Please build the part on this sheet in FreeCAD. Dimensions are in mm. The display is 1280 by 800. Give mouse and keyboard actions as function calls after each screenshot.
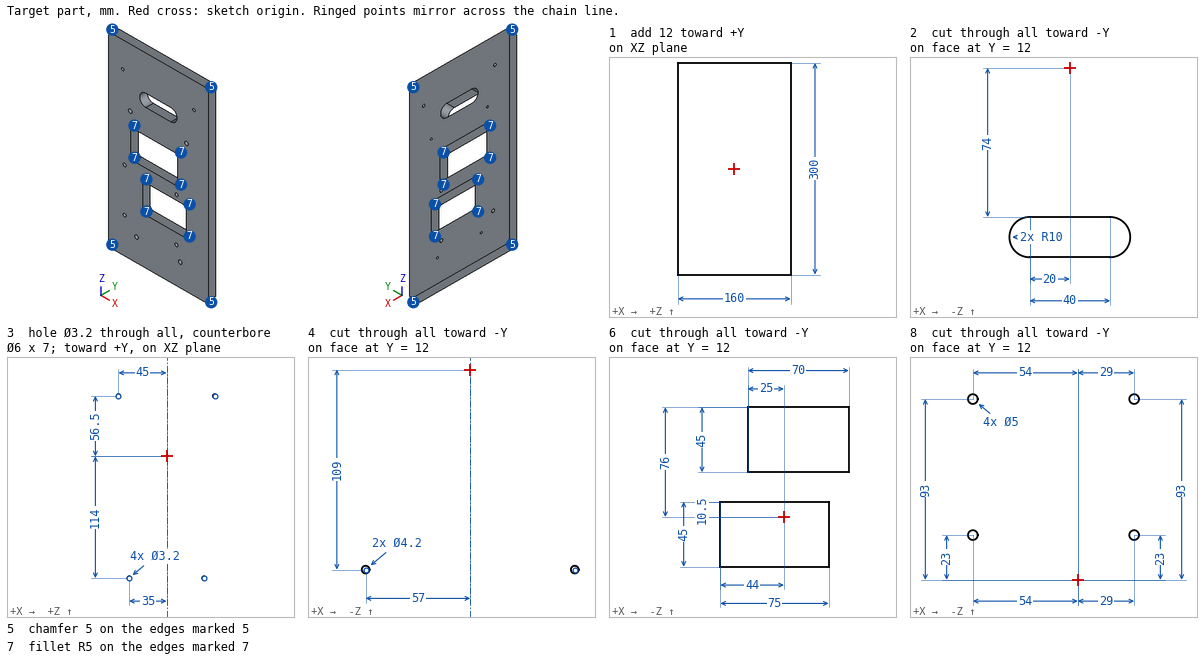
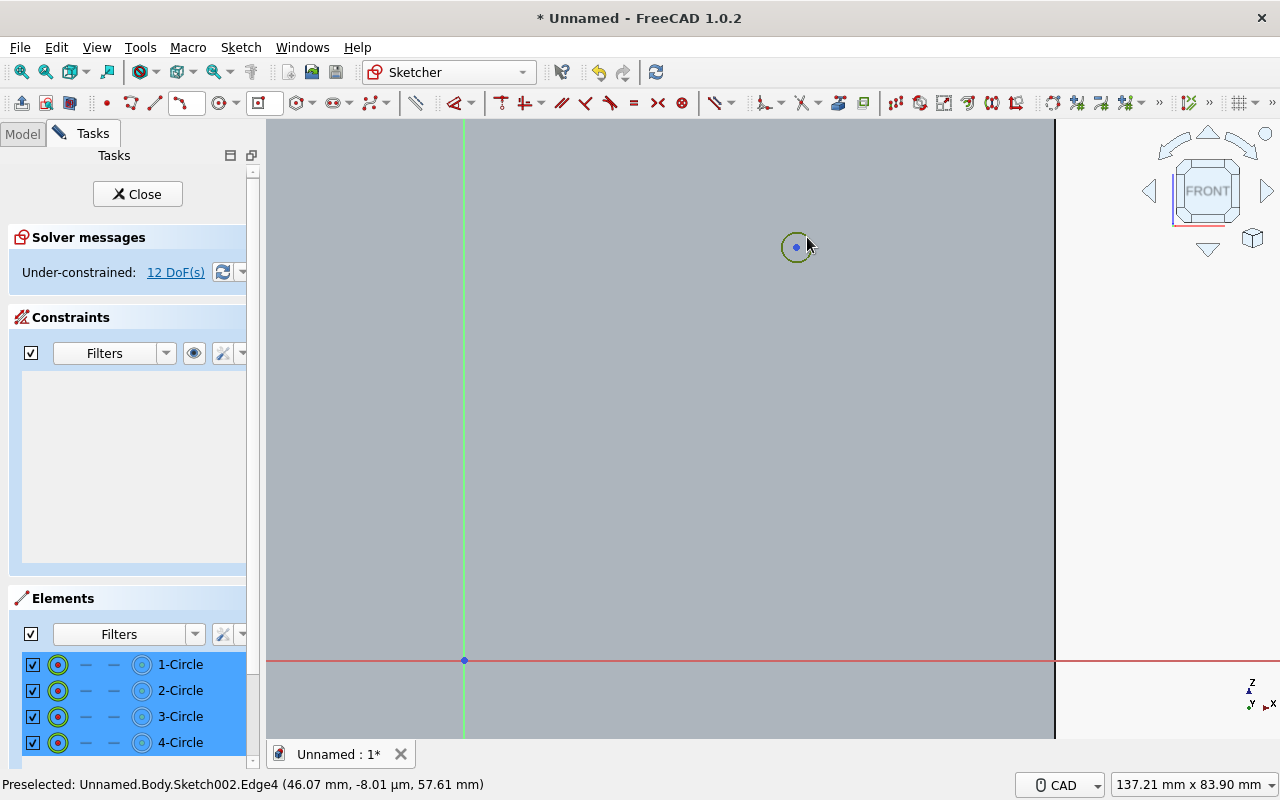
click(634, 104)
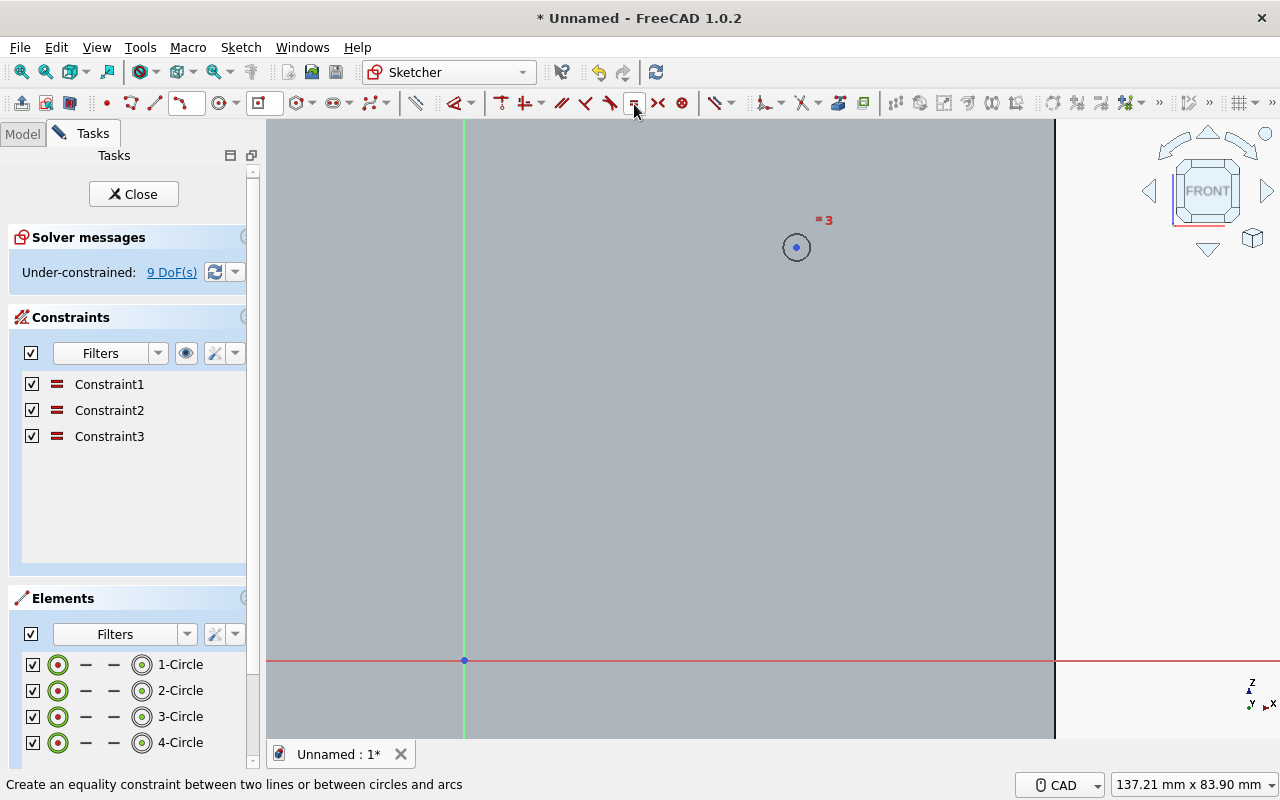
scroll(808, 238, down, 6)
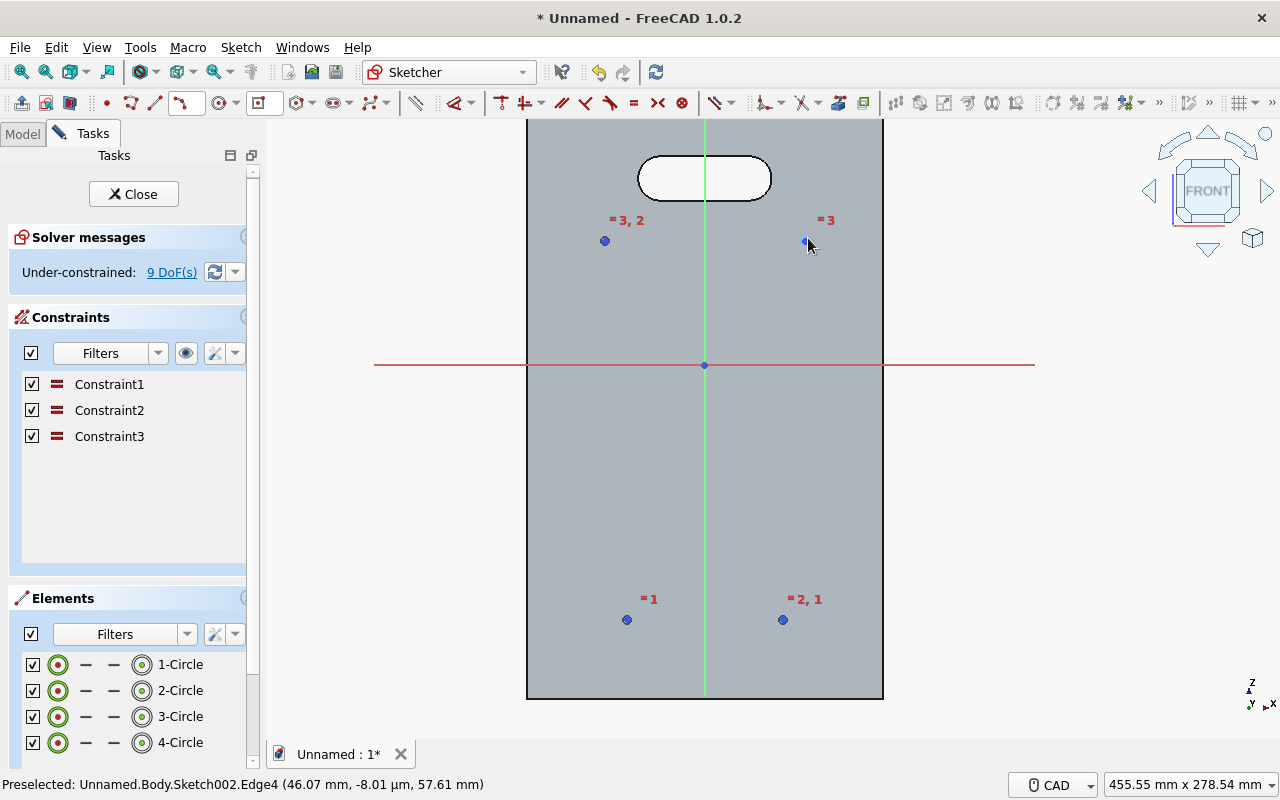
click(627, 620)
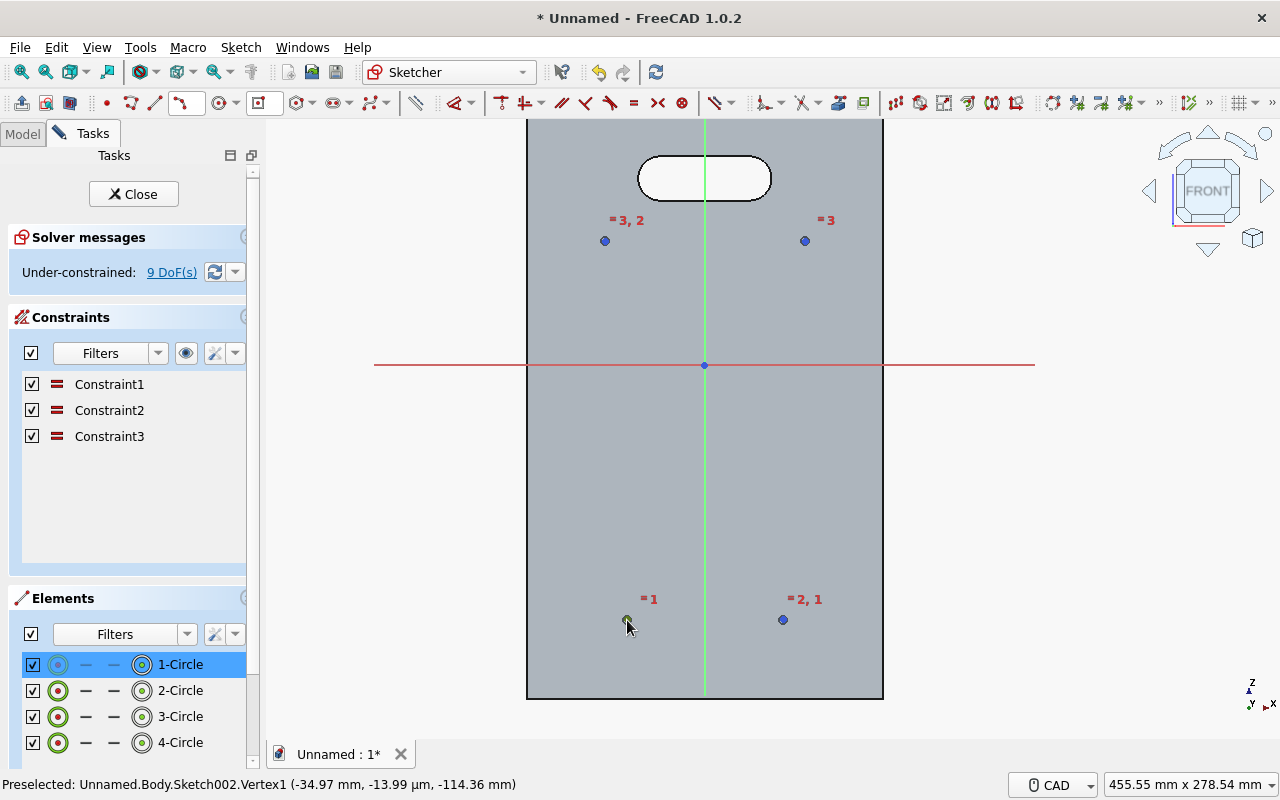
click(783, 620)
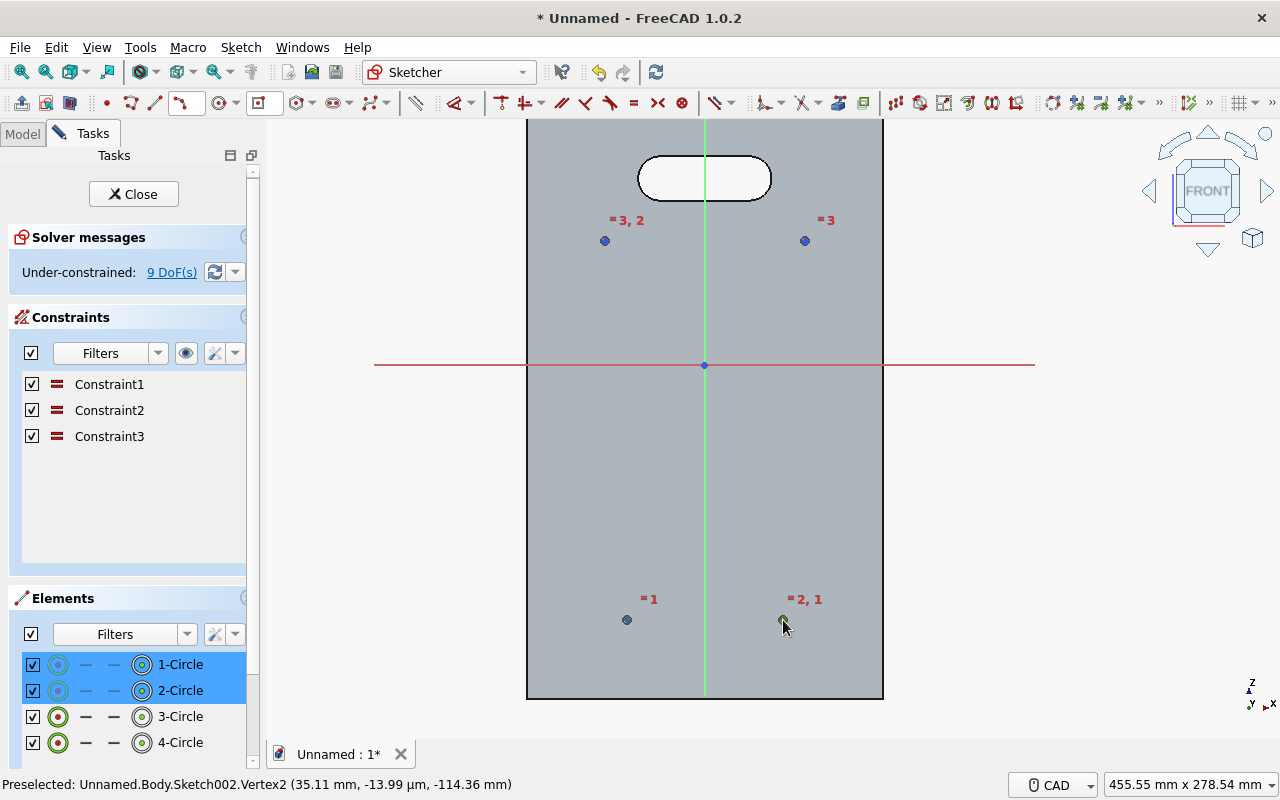
click(705, 671)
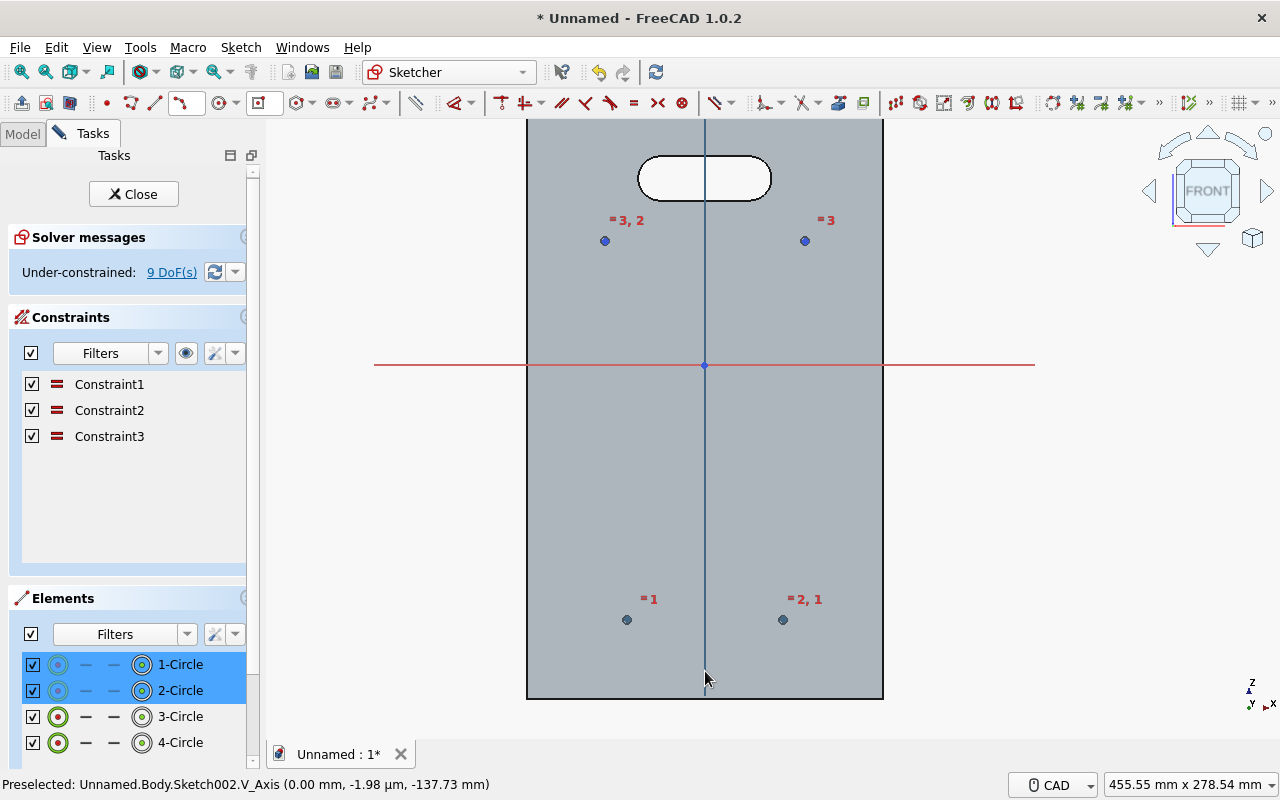
click(658, 104)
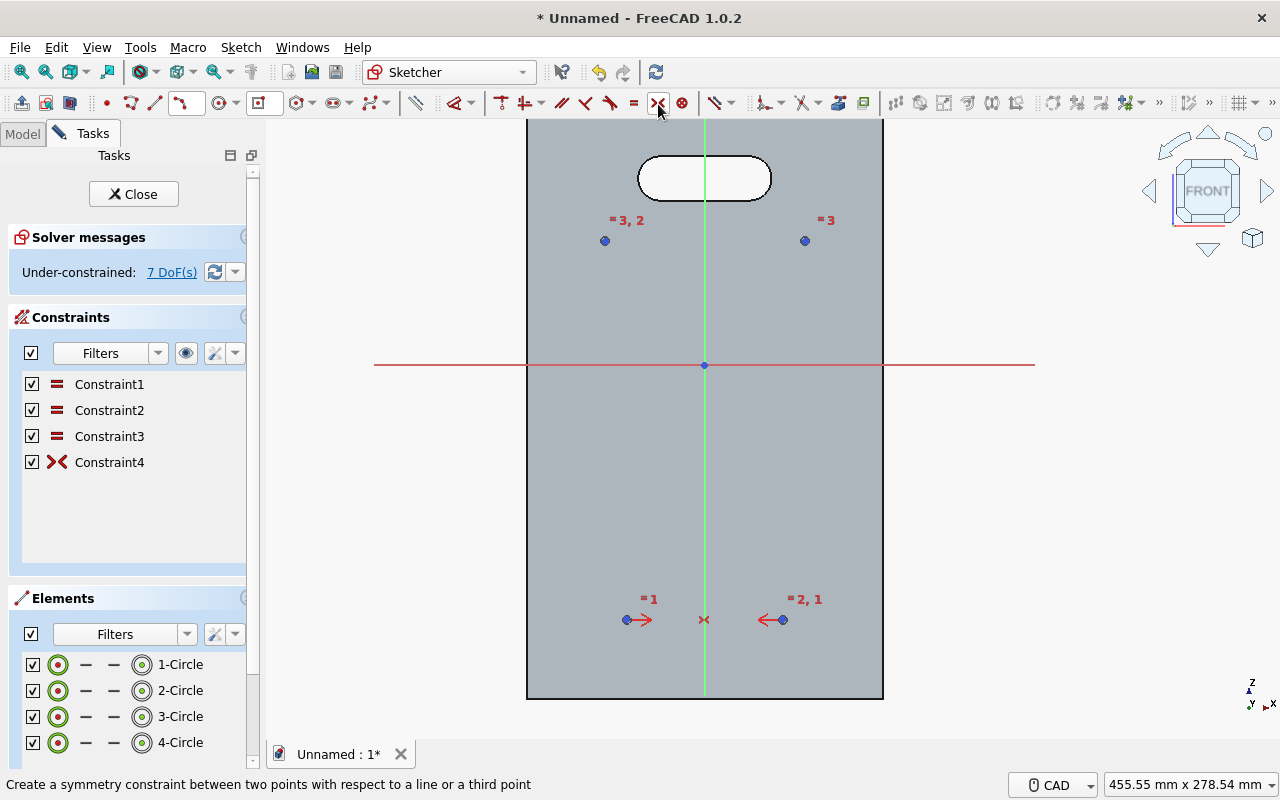
click(605, 241)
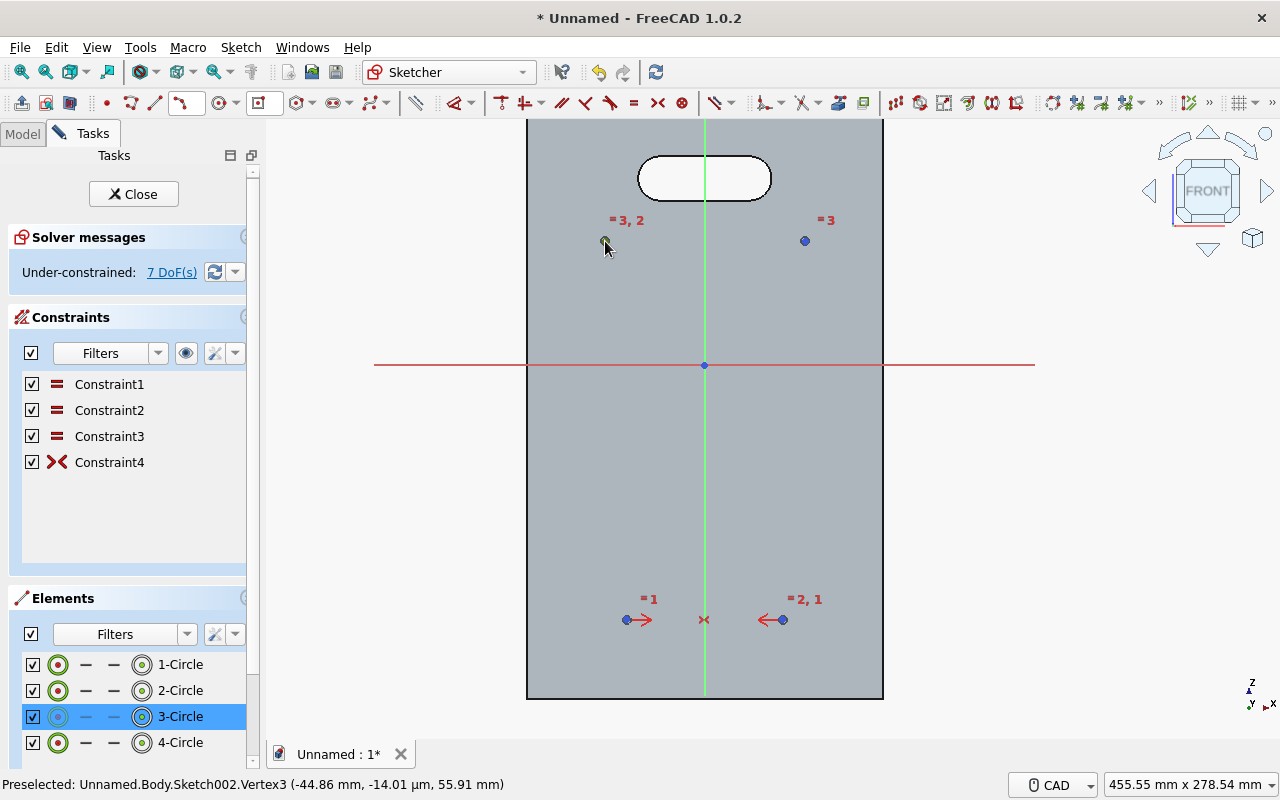
click(805, 241)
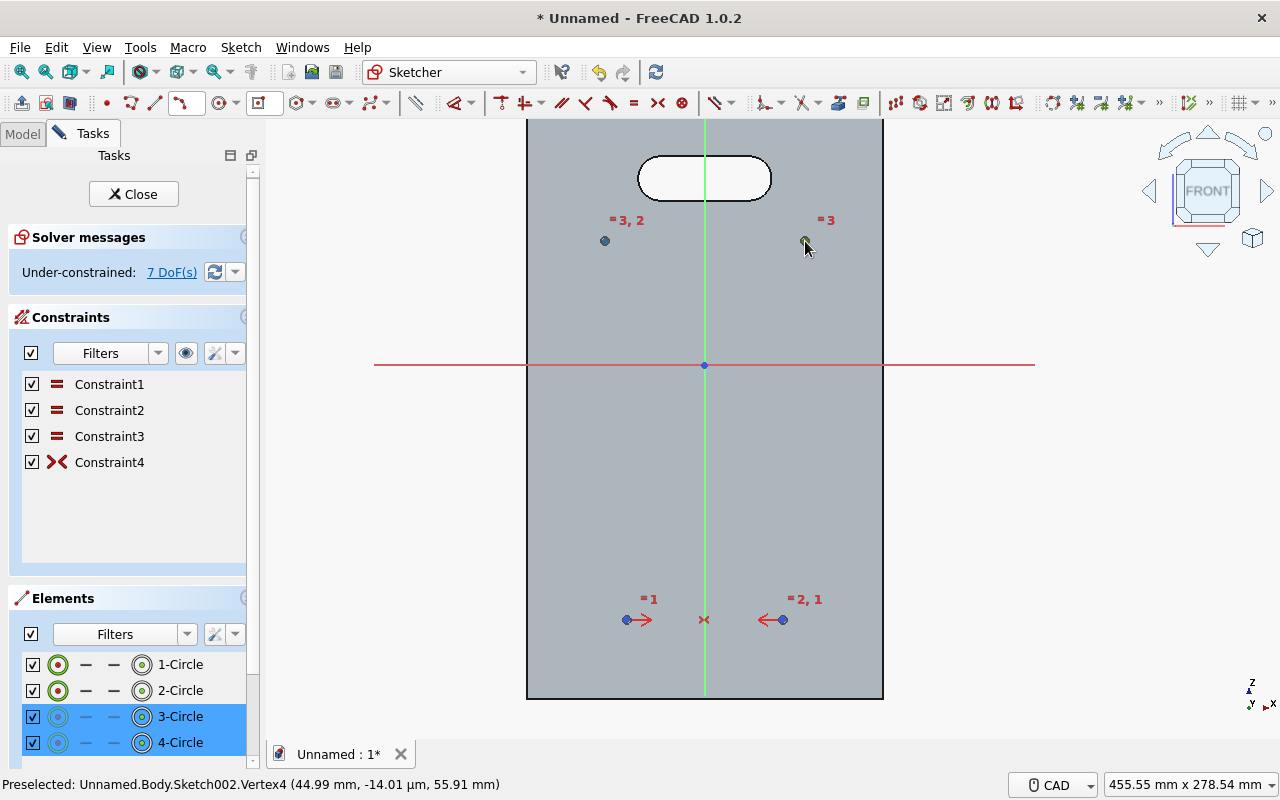
click(705, 671)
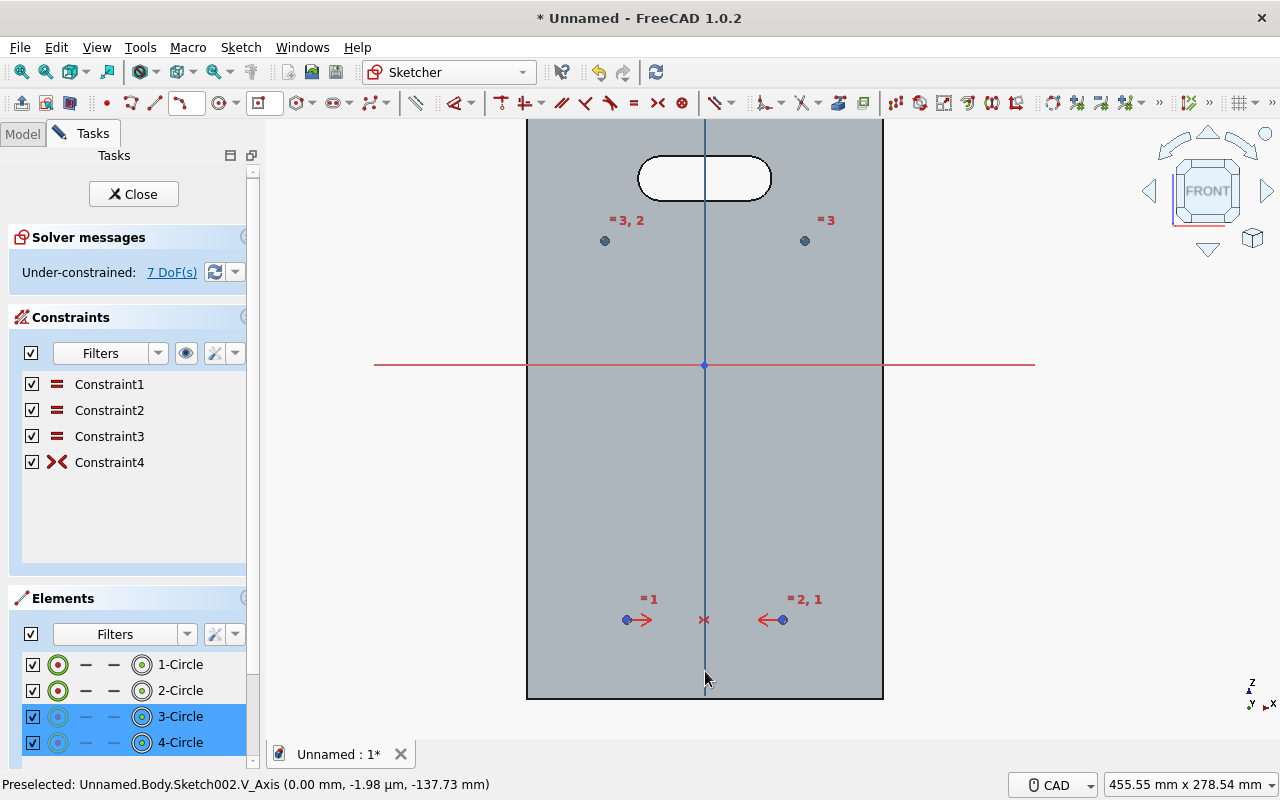
click(658, 104)